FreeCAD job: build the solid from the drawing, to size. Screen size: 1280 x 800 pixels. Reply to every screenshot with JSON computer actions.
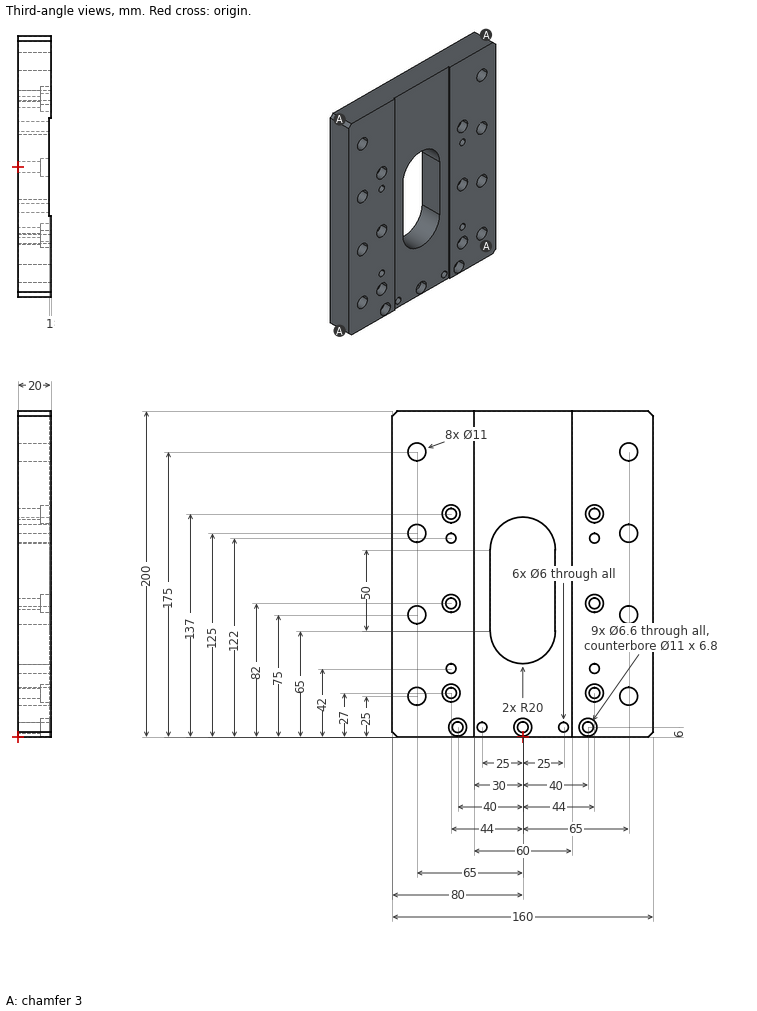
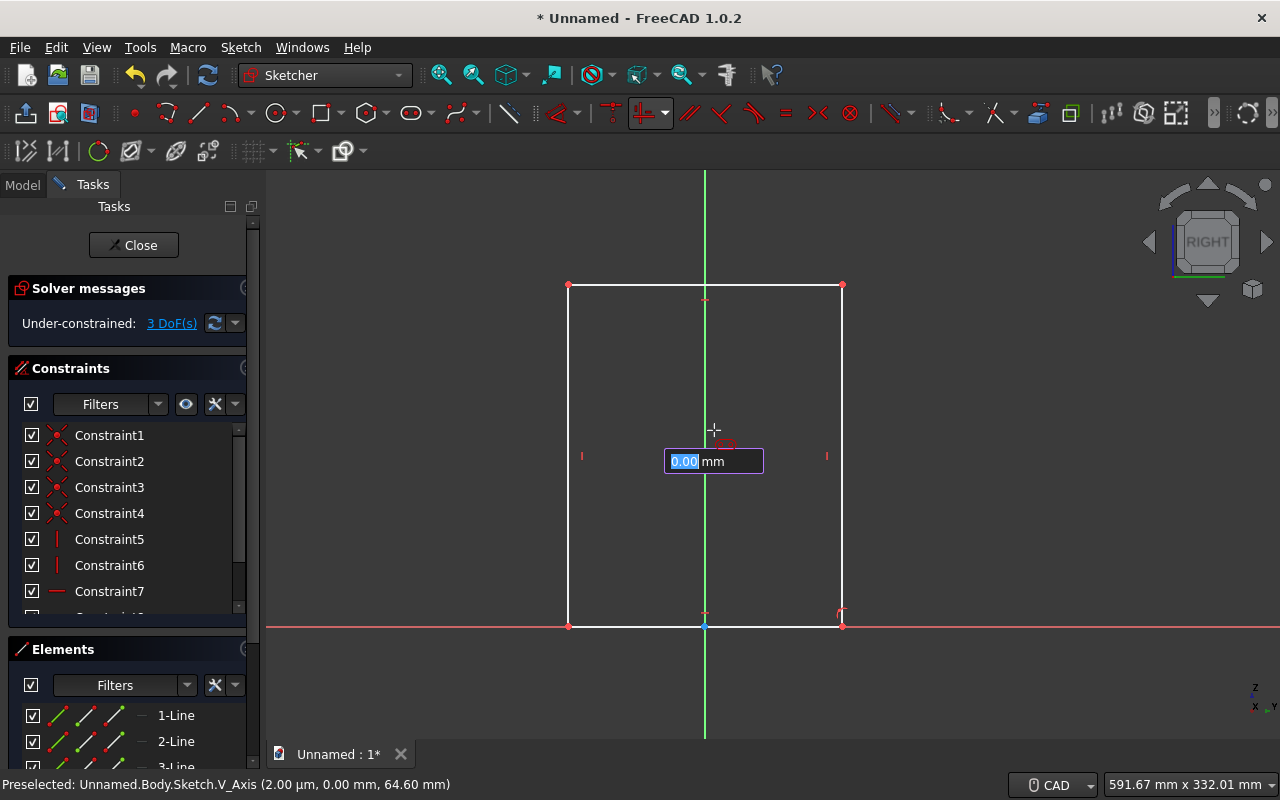
{"action": "left_click", "coordinate": [671, 472]}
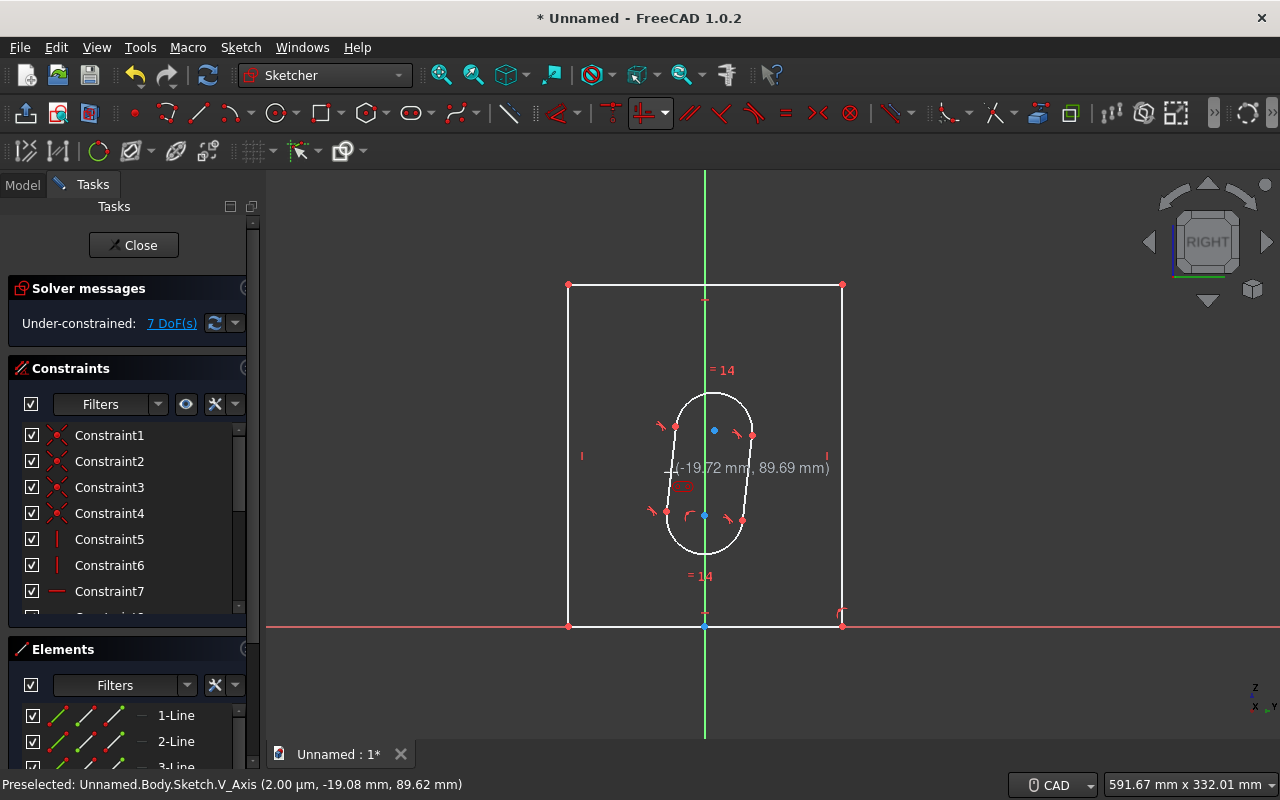
{"action": "left_click", "coordinate": [276, 114]}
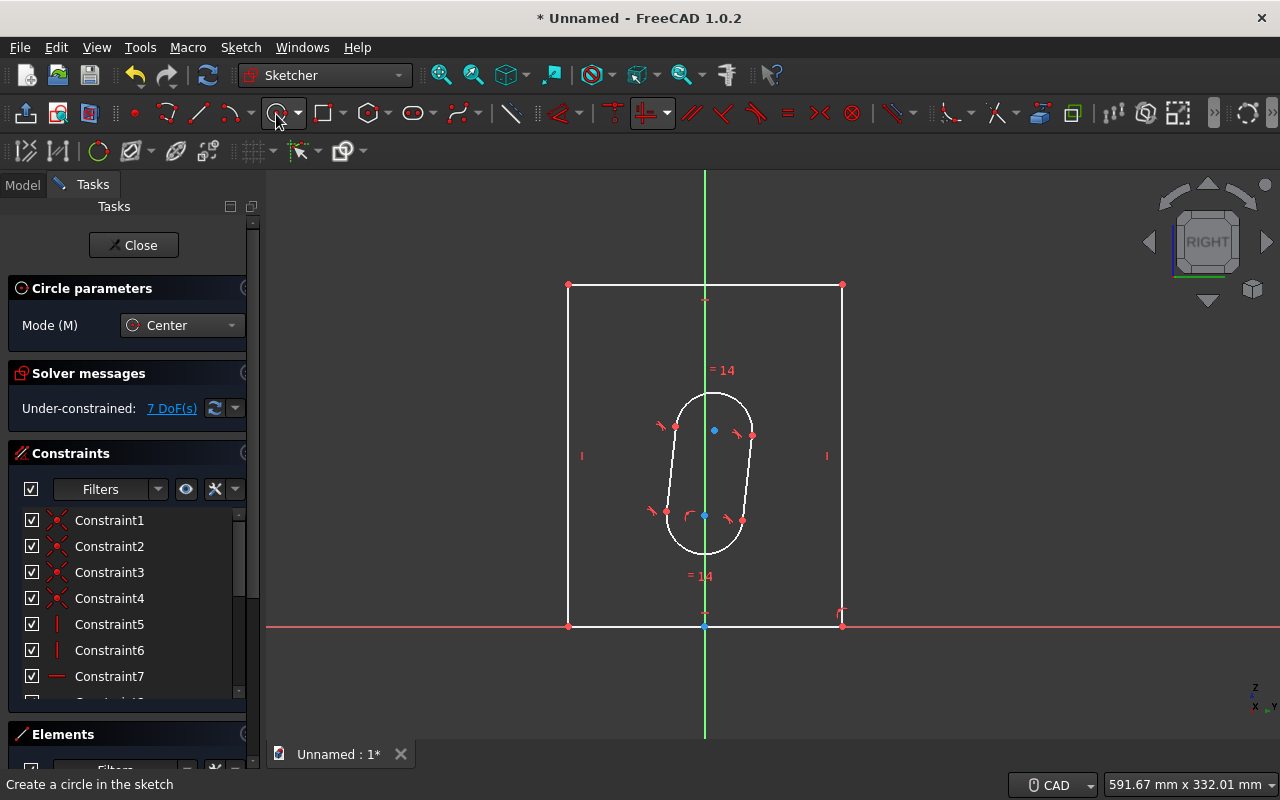
{"action": "scroll", "coordinate": [593, 327], "scroll_direction": "up", "scroll_amount": 5}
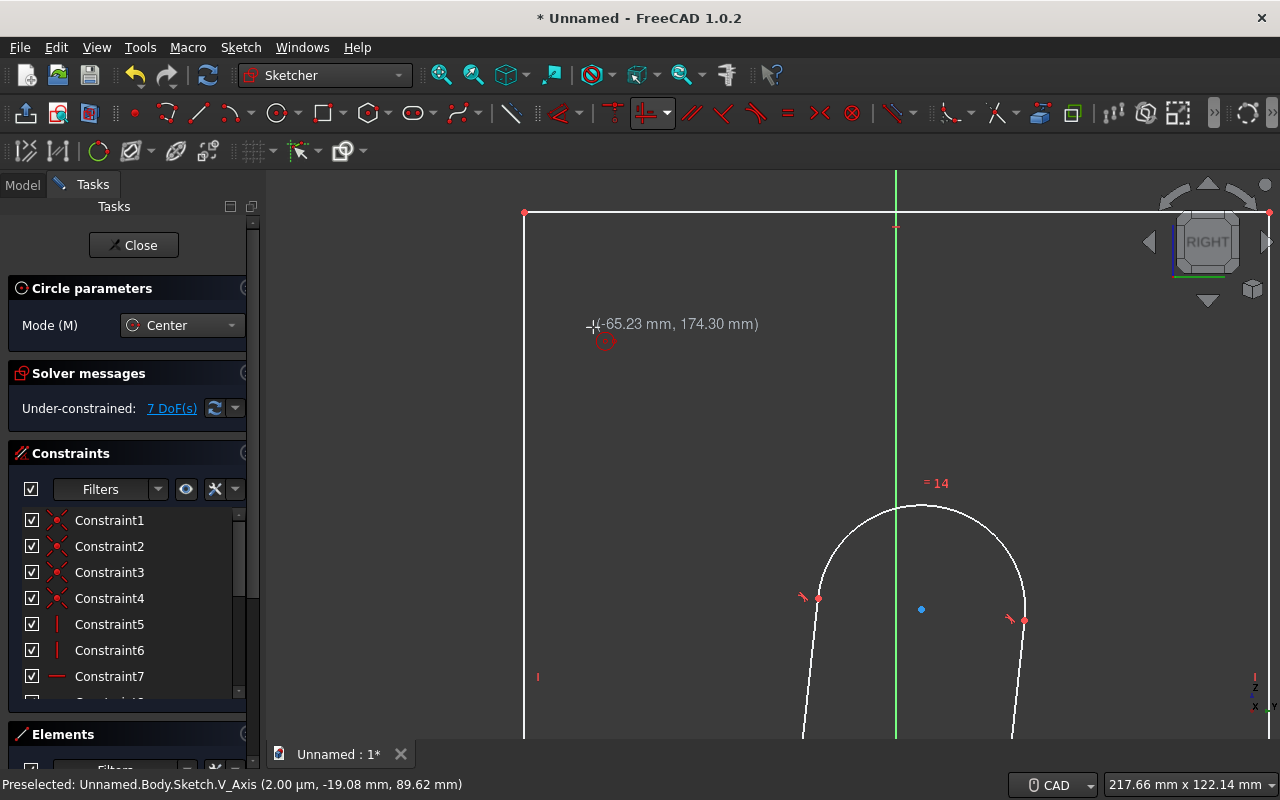
{"action": "left_click", "coordinate": [594, 326]}
{"action": "mouse_move", "coordinate": [612, 308]}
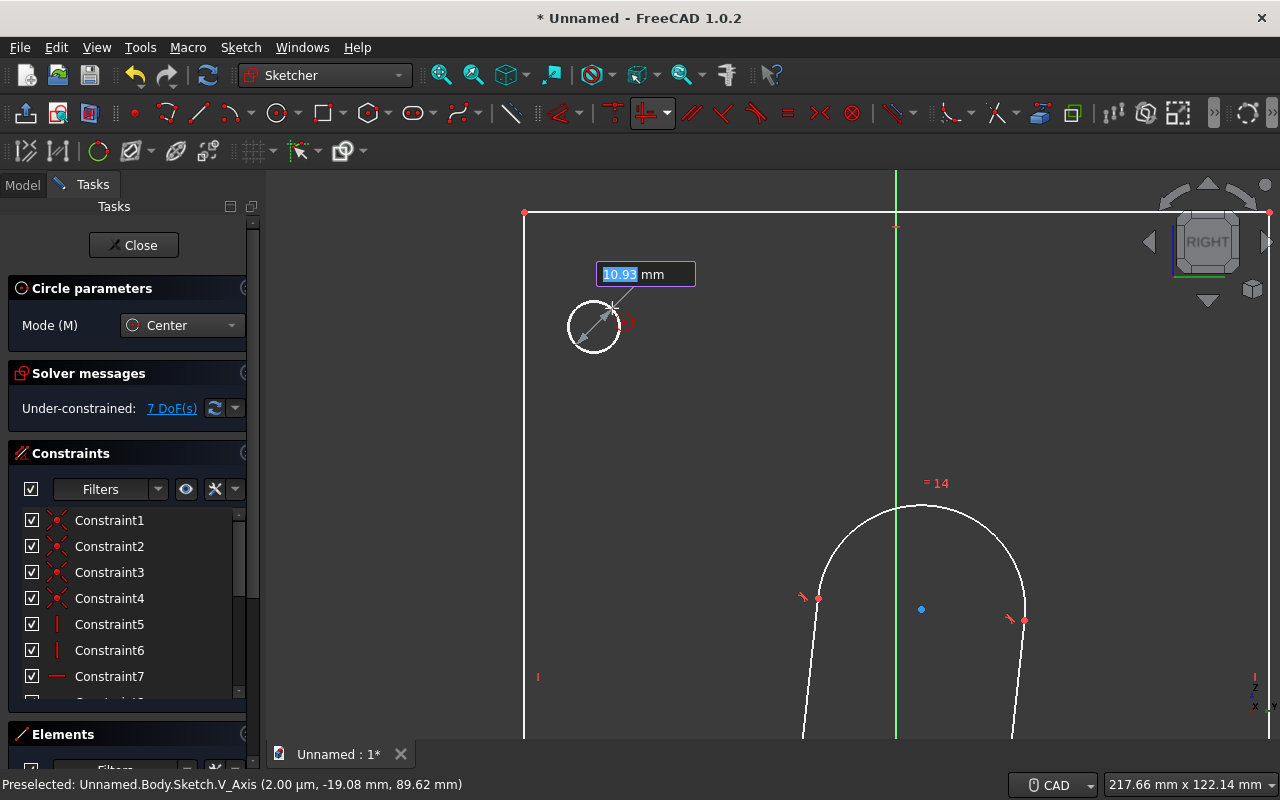
{"action": "type", "text": "11"}
{"action": "key", "text": "Return"}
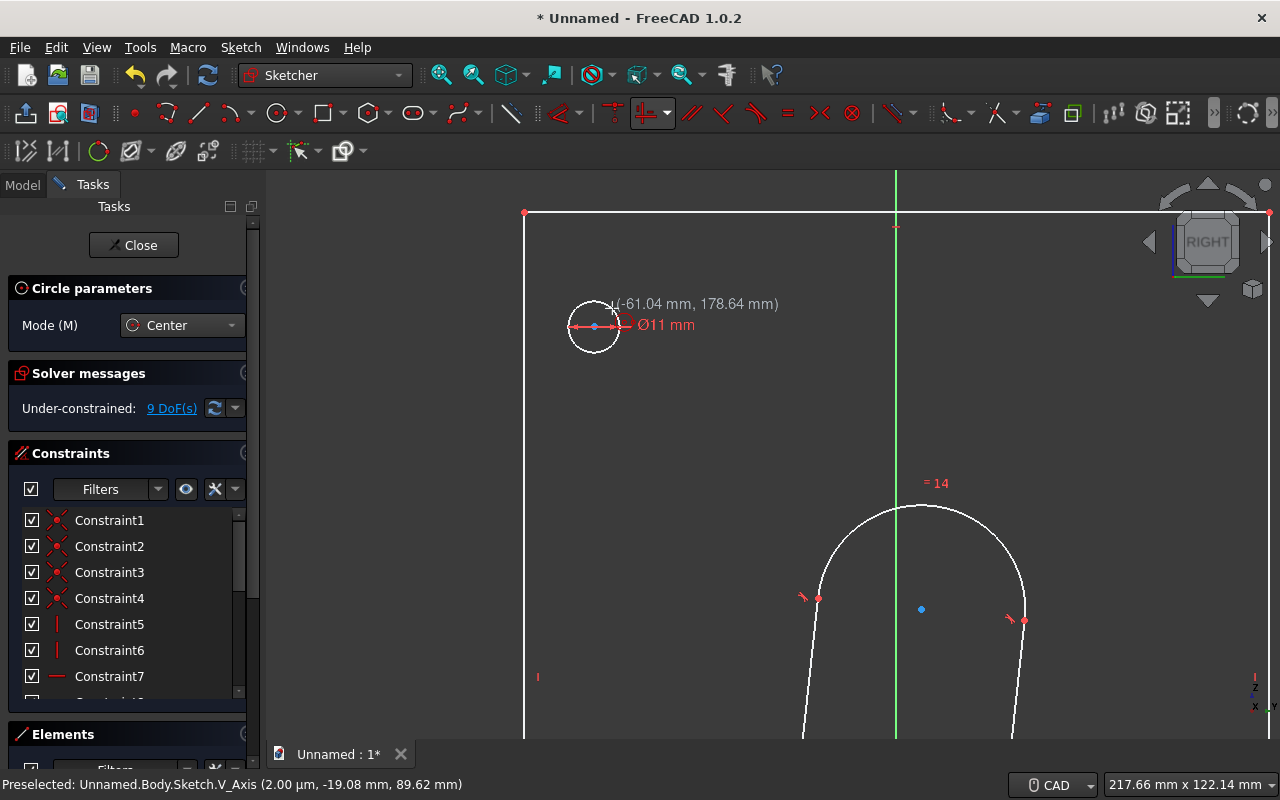
{"action": "left_click", "coordinate": [594, 559]}
{"action": "mouse_move", "coordinate": [612, 541]}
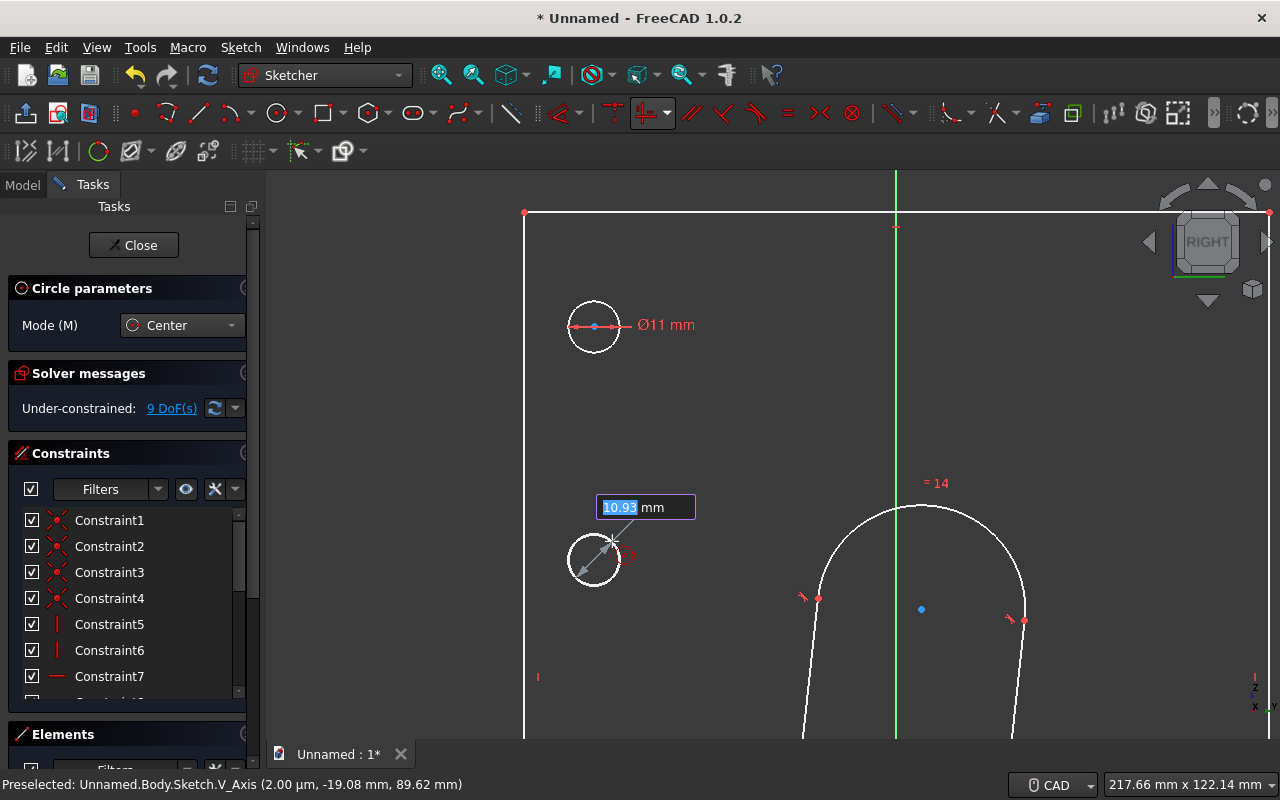
{"action": "type", "text": "11"}
{"action": "key", "text": "Return"}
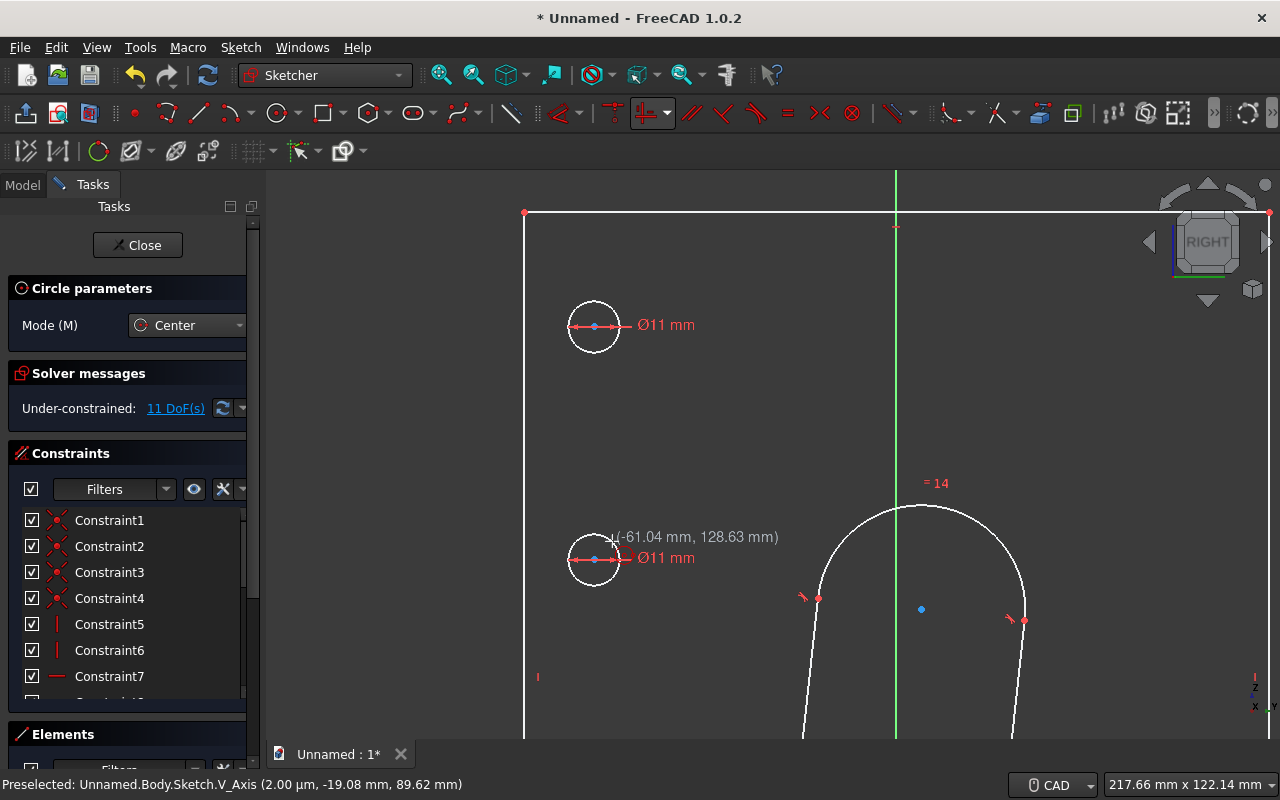
{"action": "scroll", "coordinate": [593, 326], "scroll_direction": "down", "scroll_amount": 5}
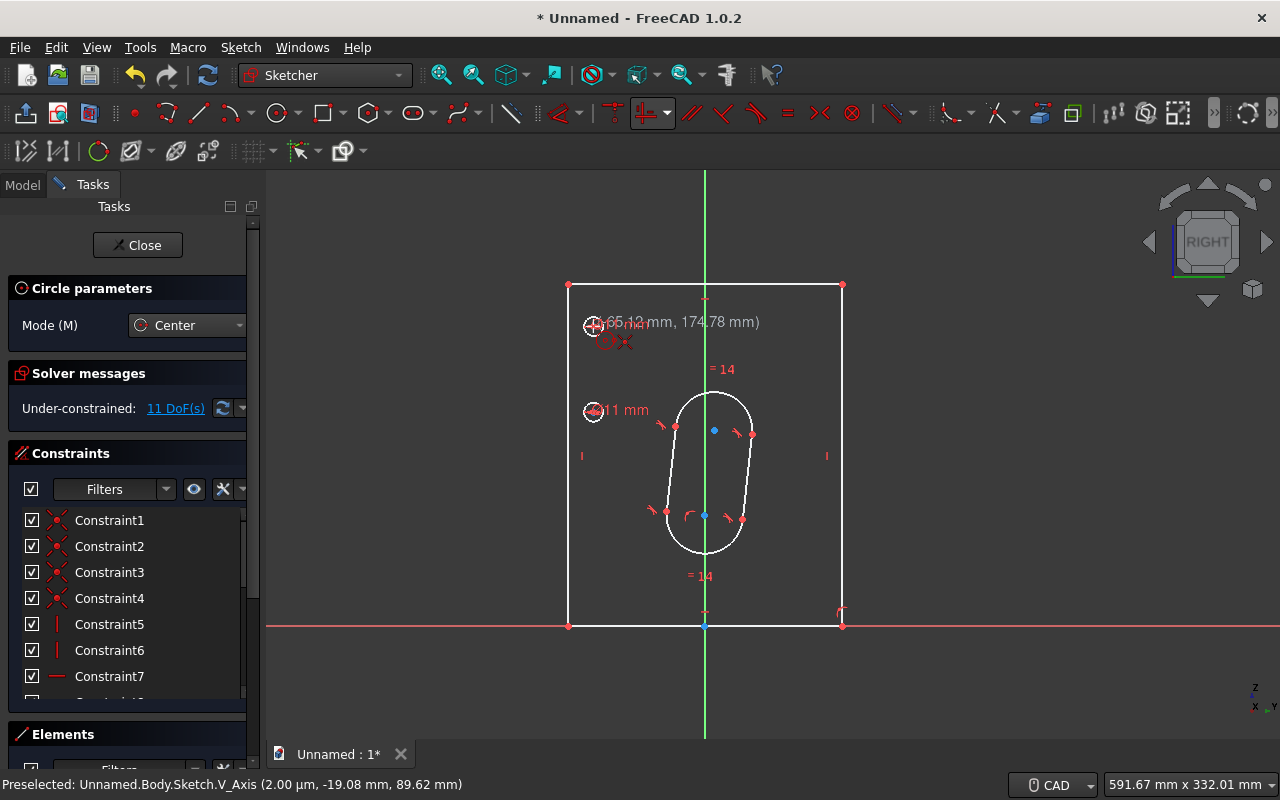
{"action": "scroll", "coordinate": [593, 498], "scroll_direction": "up", "scroll_amount": 5}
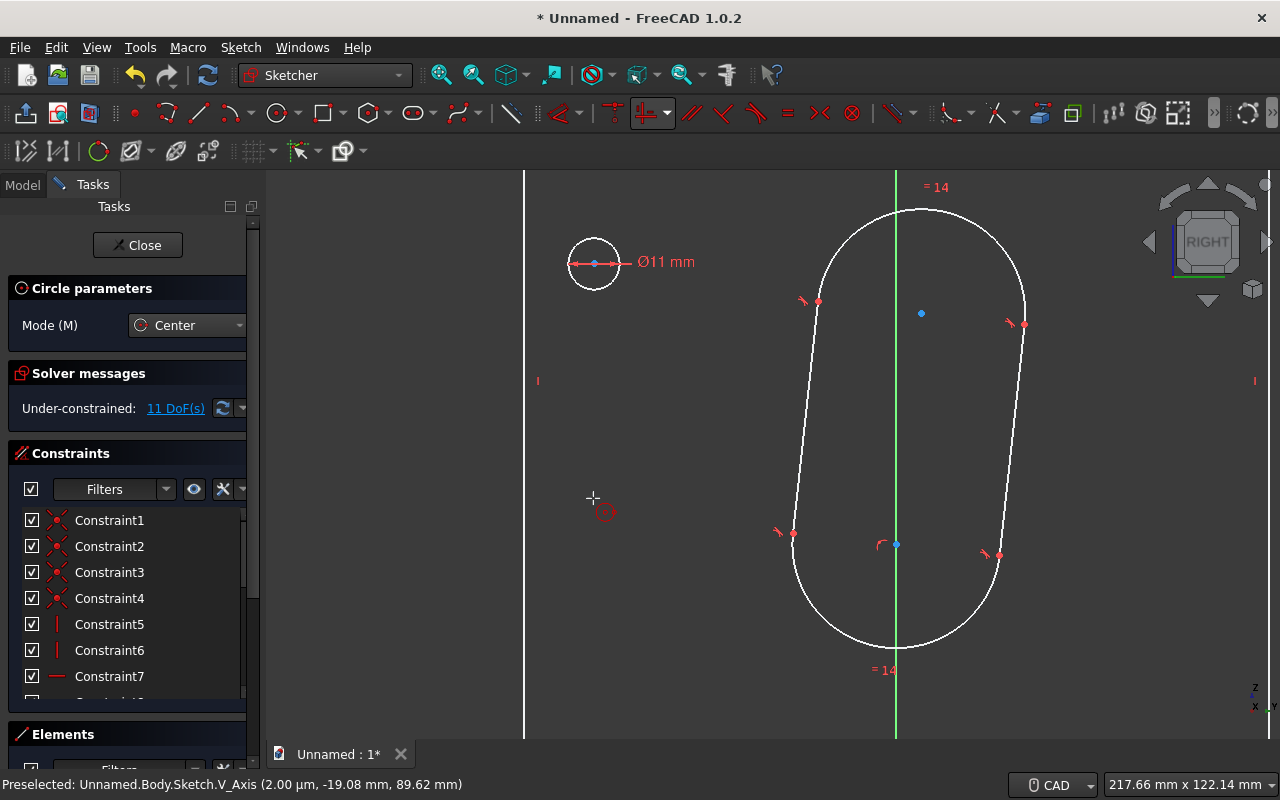
{"action": "left_click", "coordinate": [594, 496]}
{"action": "mouse_move", "coordinate": [612, 478]}